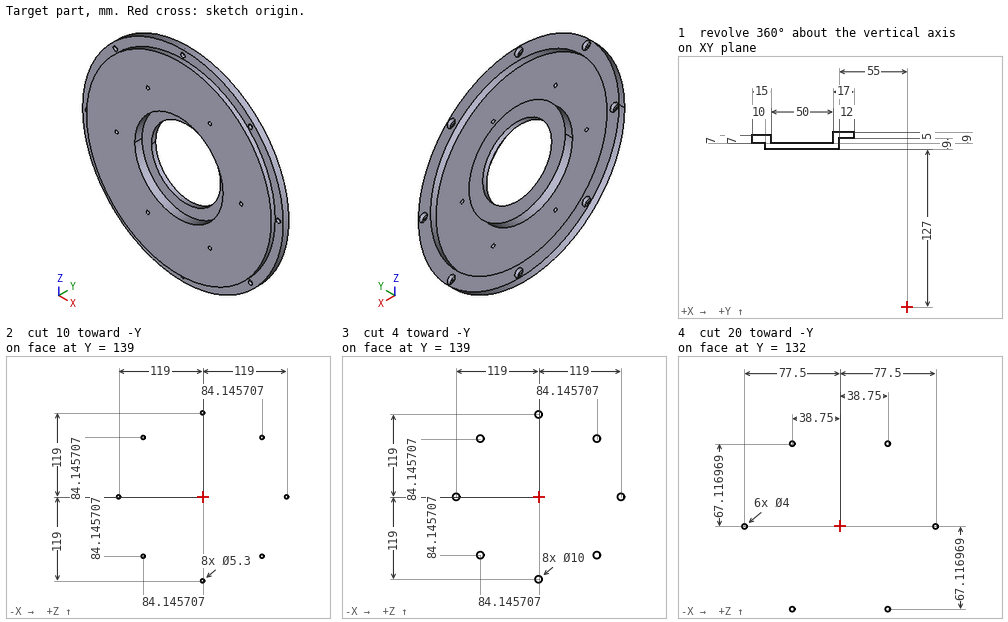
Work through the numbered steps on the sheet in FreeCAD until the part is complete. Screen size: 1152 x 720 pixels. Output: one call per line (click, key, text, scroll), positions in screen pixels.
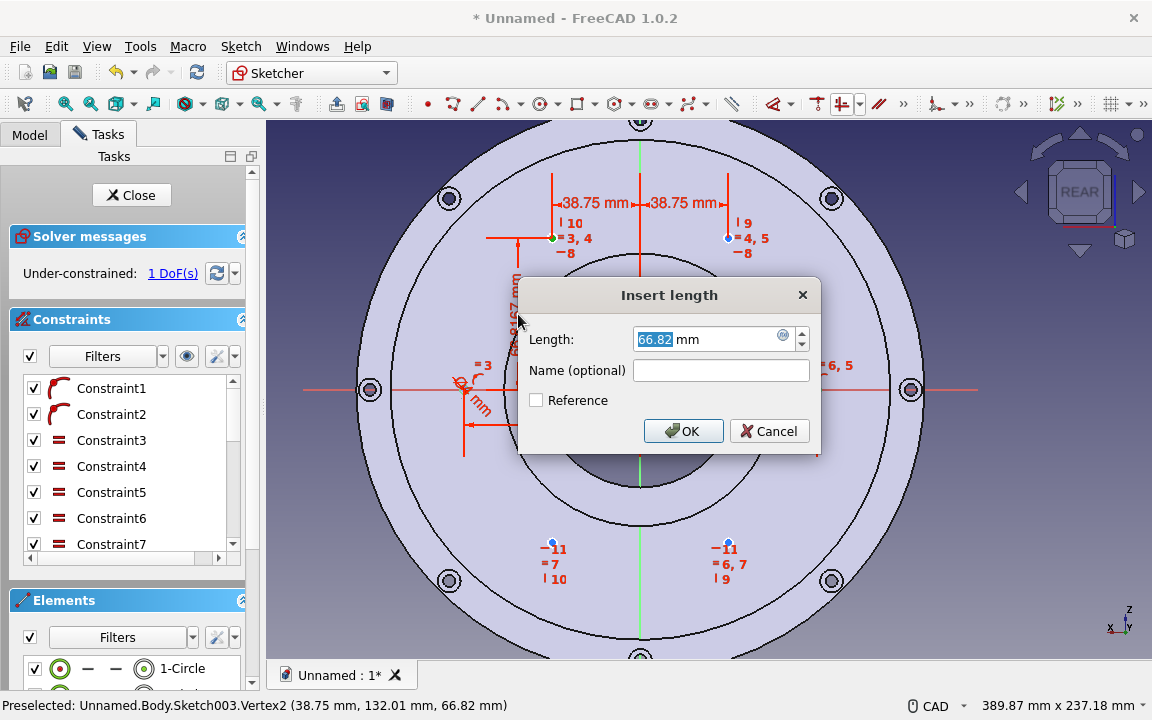
text(67.116969)
key(Return)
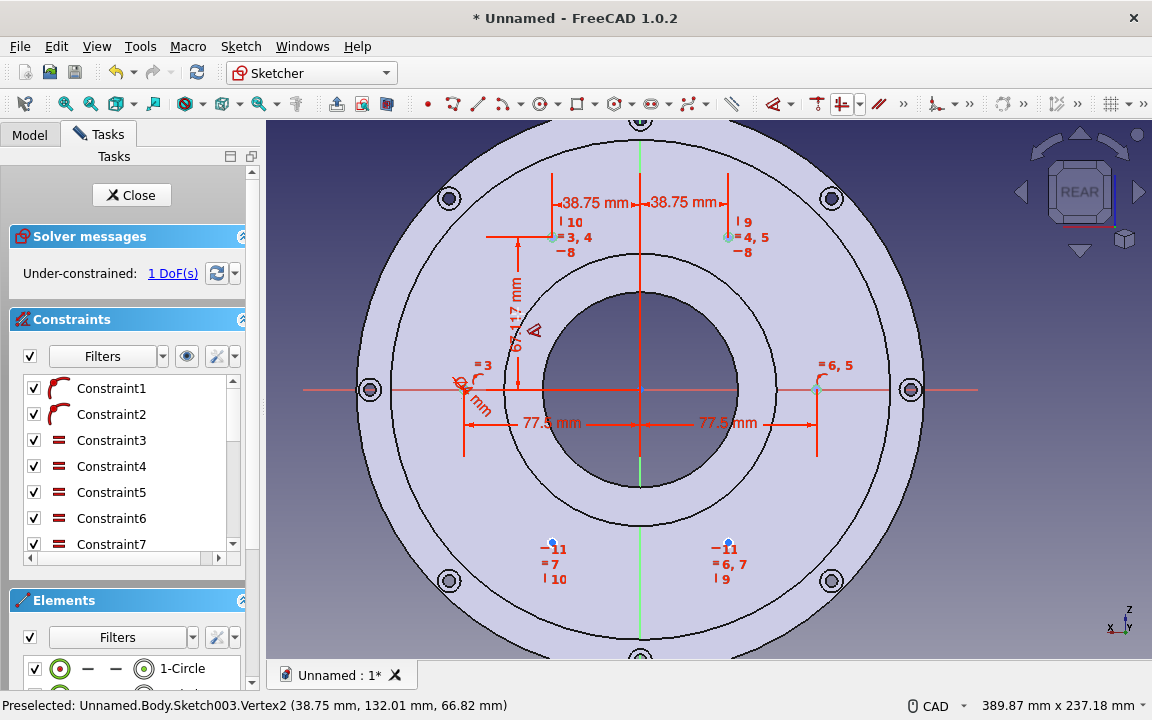
click(728, 543)
click(762, 466)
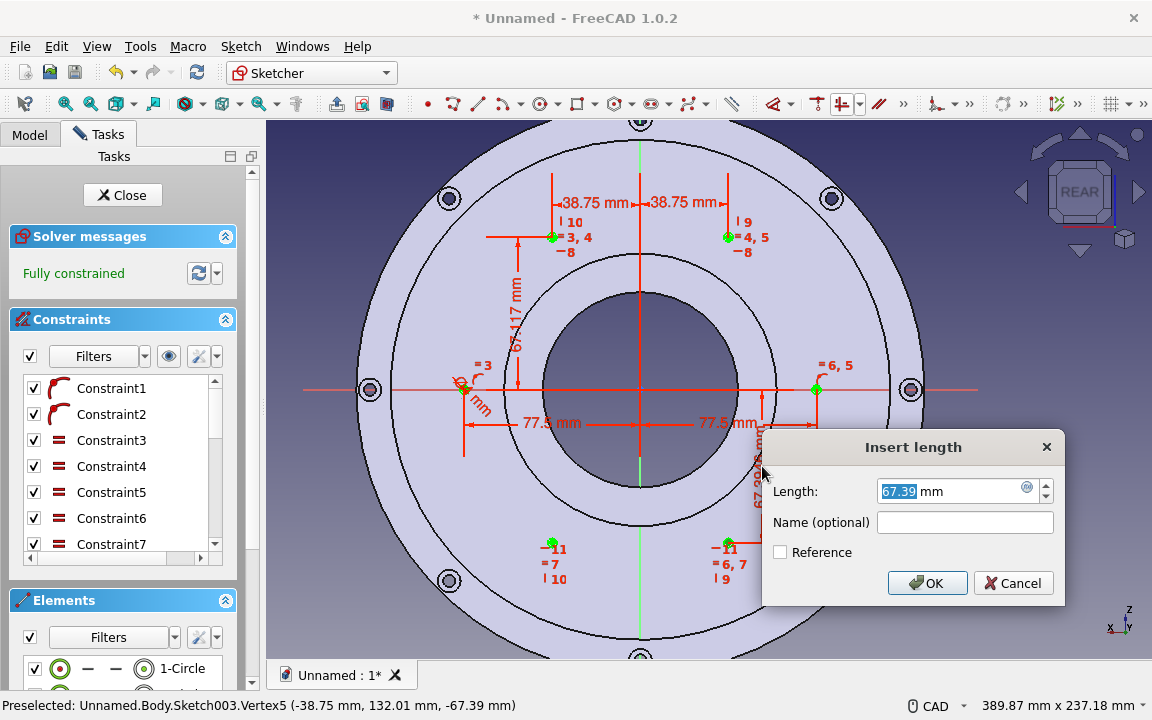
text(67.116969)
key(Return)
key(Escape)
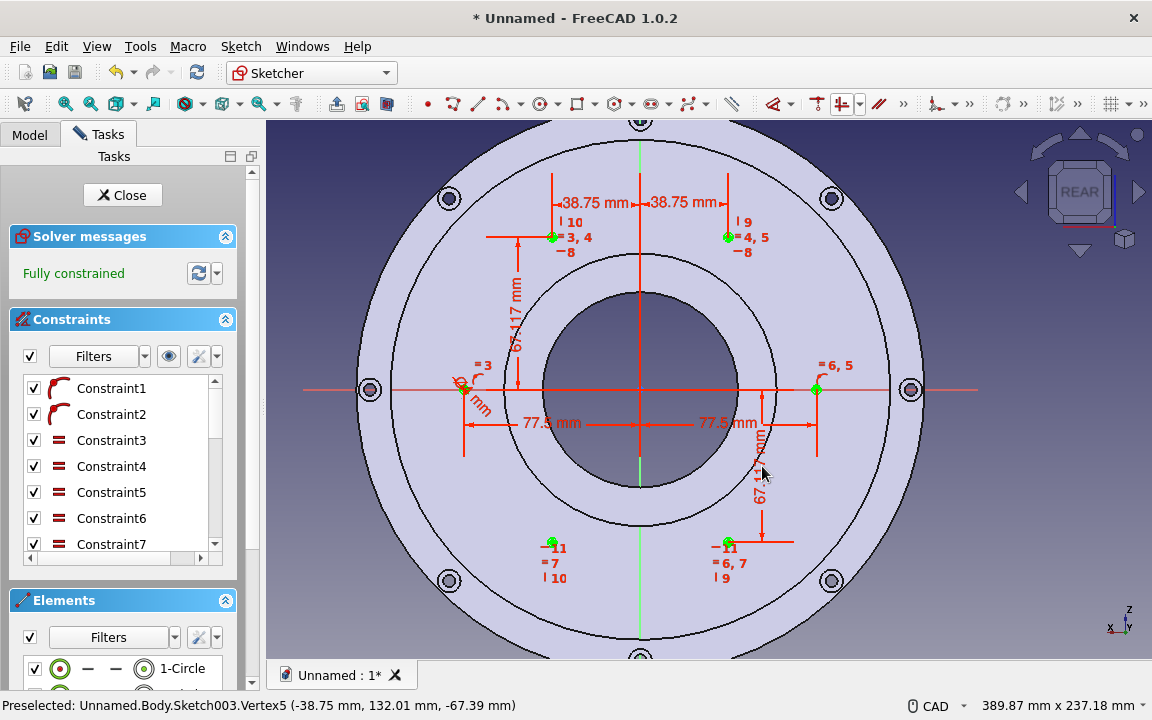
click(123, 195)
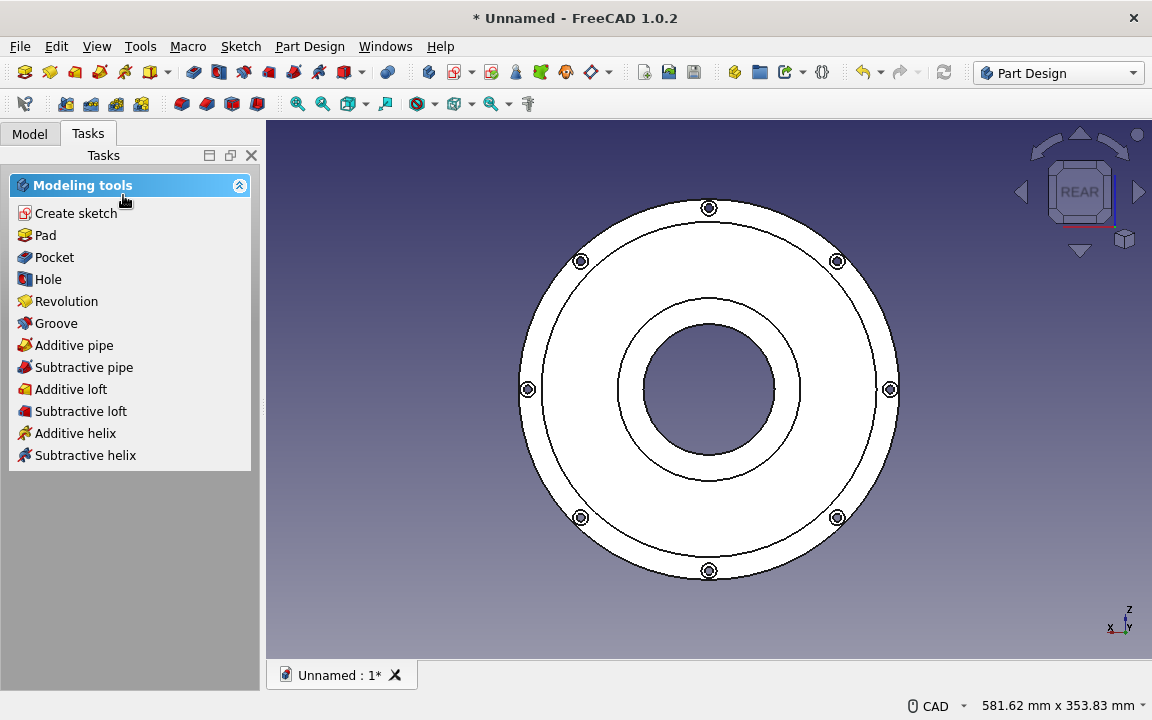
click(194, 72)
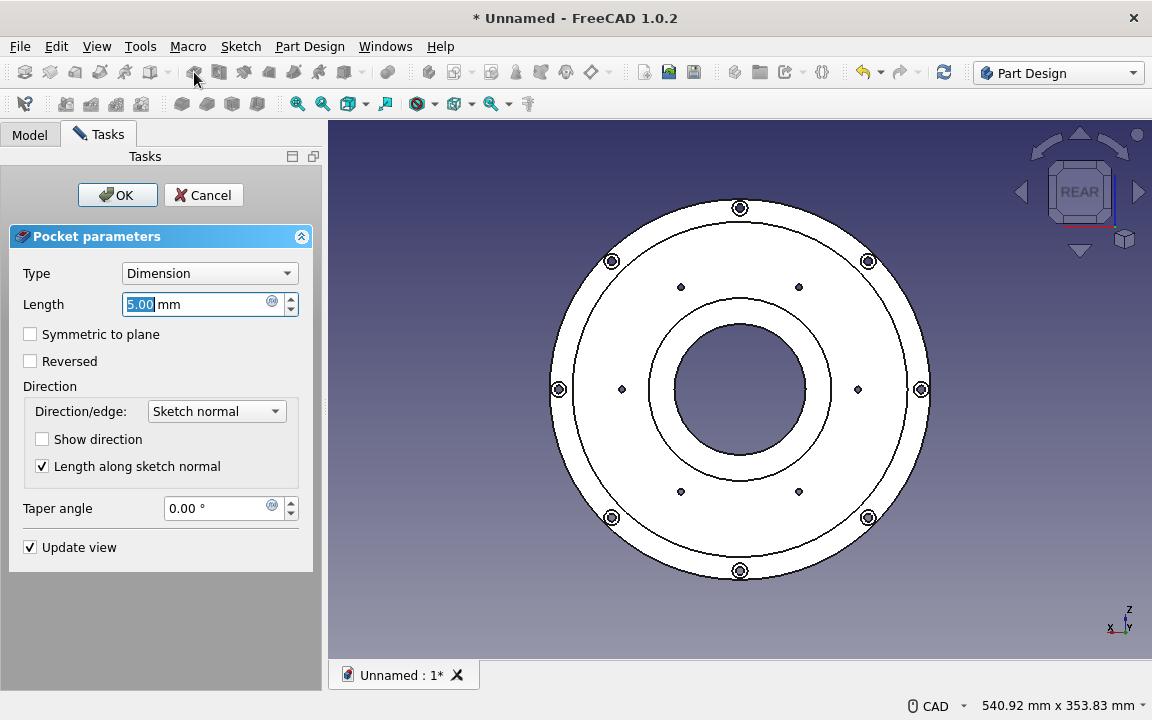
text(20)
key(Tab)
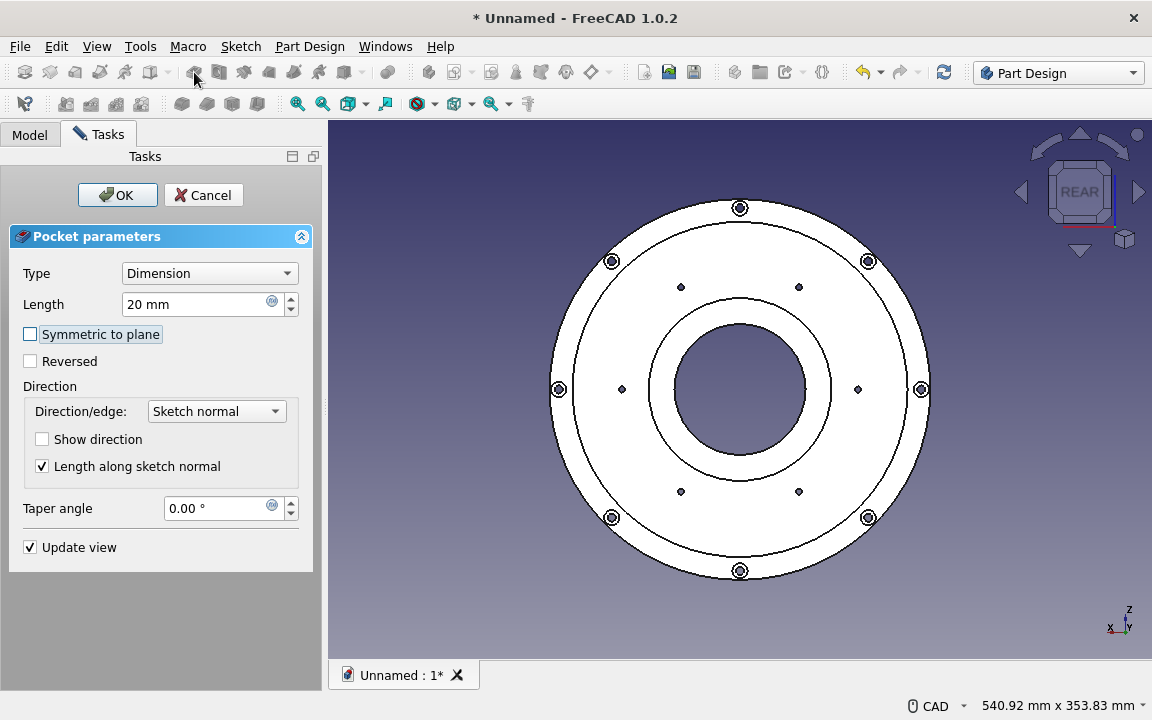
click(118, 195)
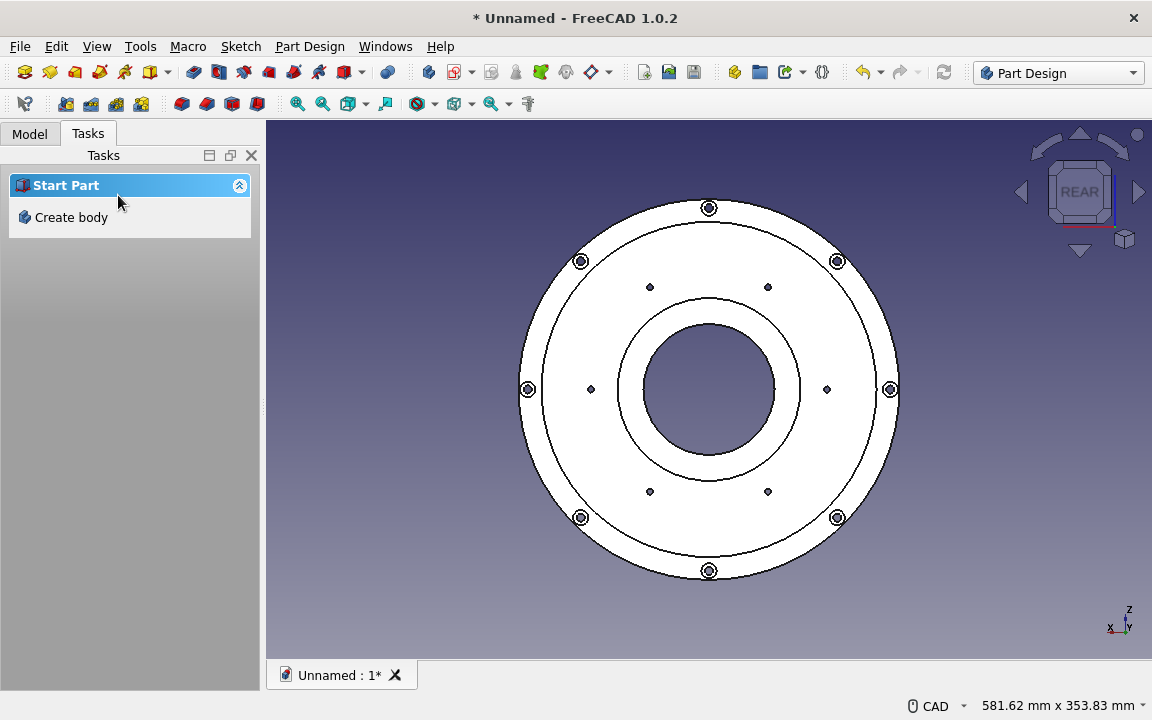
key(0)